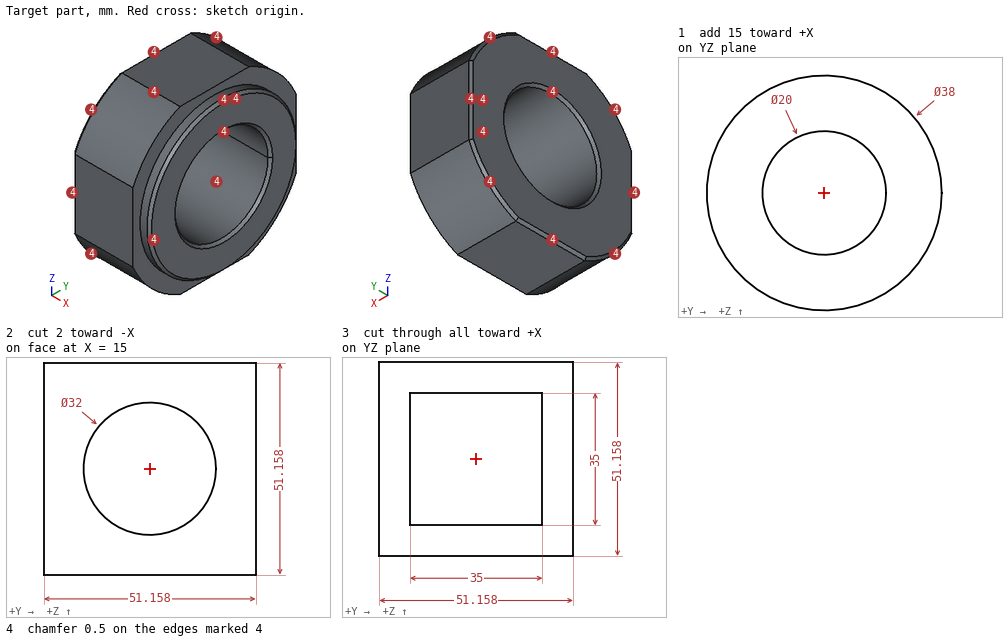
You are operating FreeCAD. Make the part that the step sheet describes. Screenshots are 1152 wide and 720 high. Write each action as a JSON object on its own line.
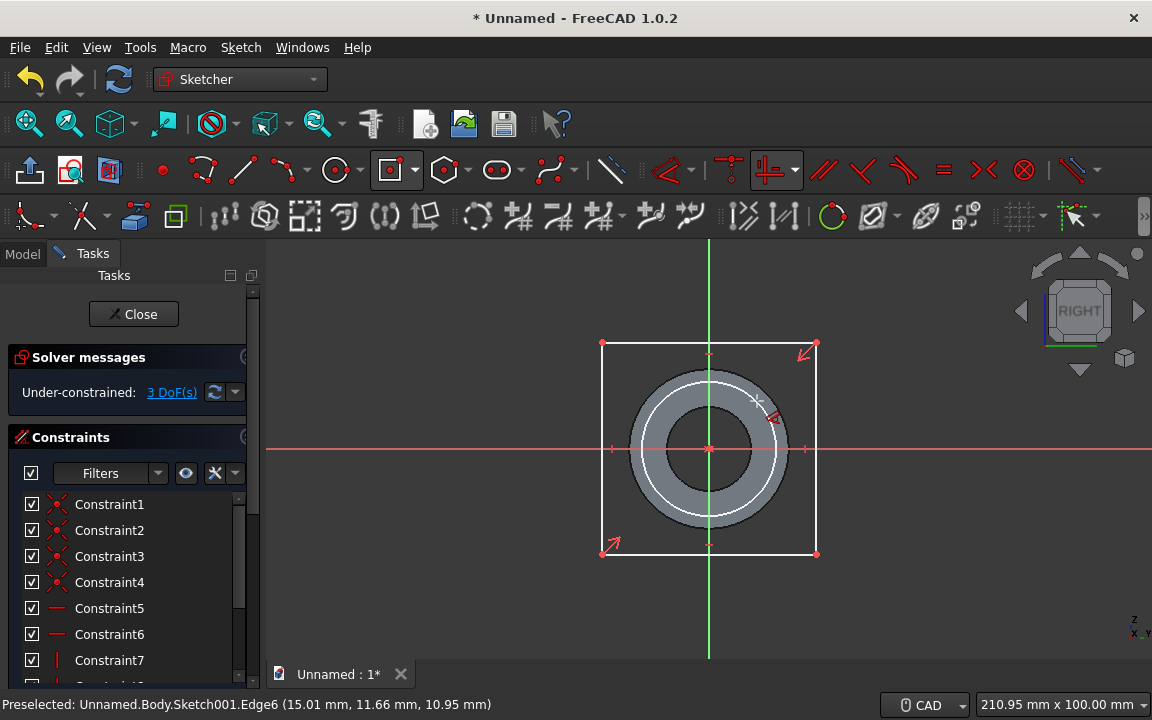
{"action": "left_click", "coordinate": [756, 401]}
{"action": "left_click", "coordinate": [778, 378]}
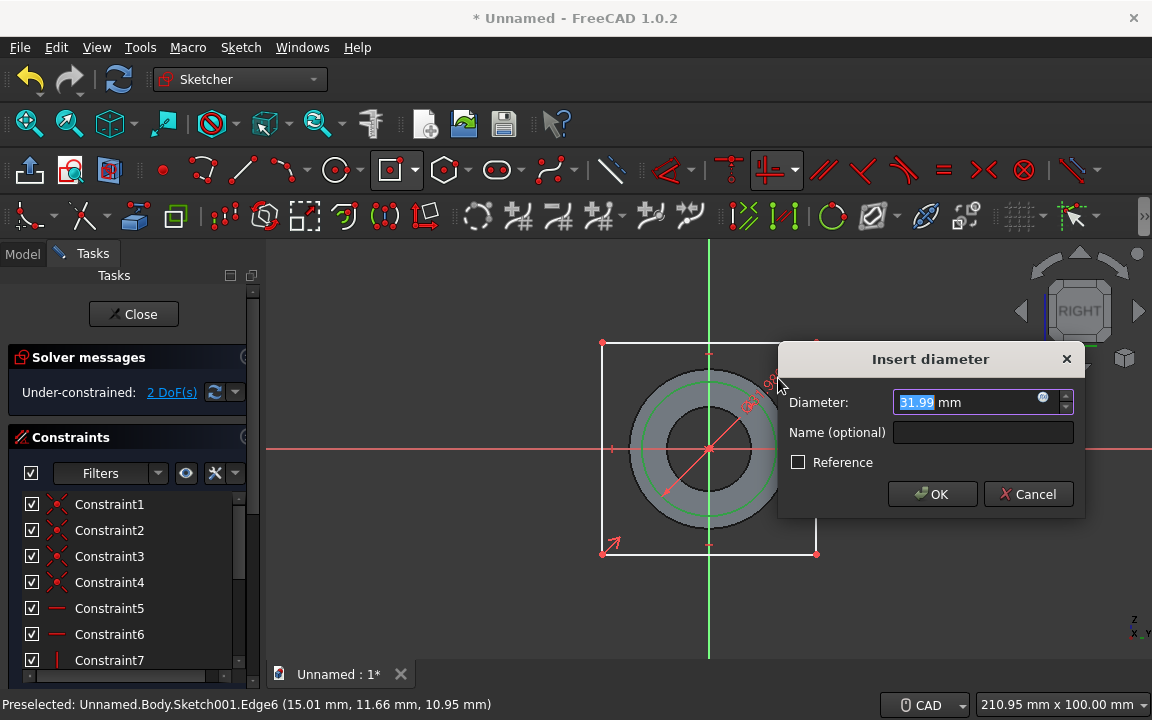
{"action": "type", "text": "32"}
{"action": "key", "text": "Return"}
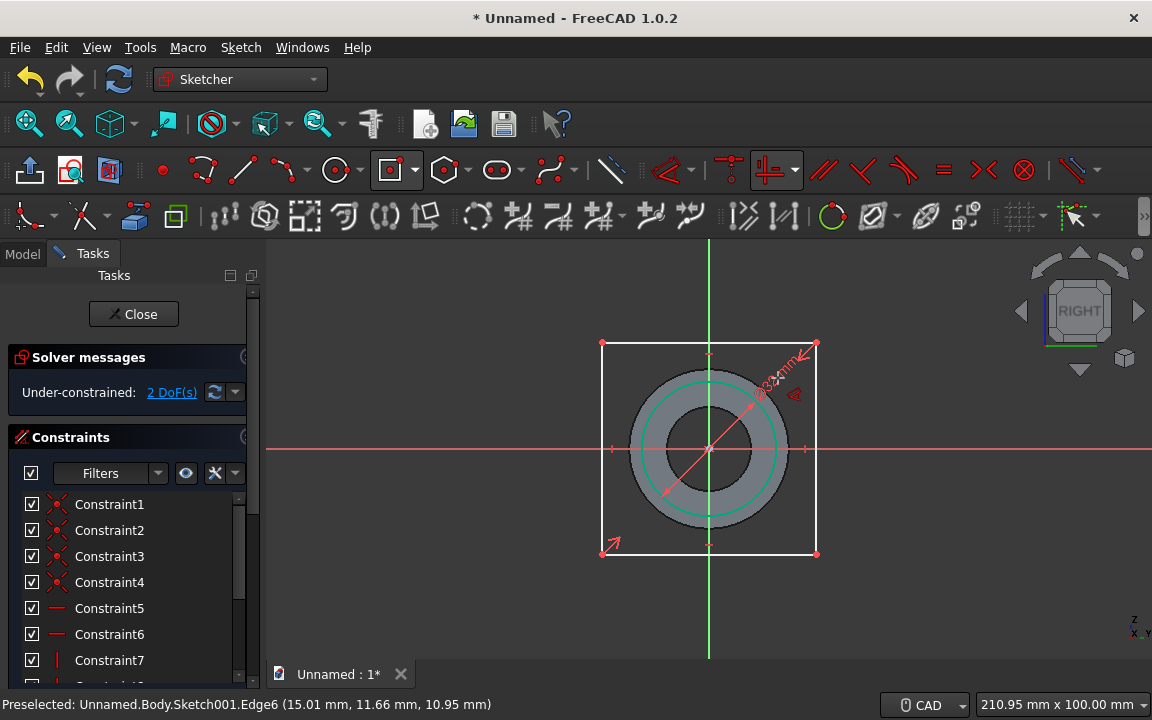
{"action": "left_click", "coordinate": [666, 555]}
{"action": "left_click", "coordinate": [660, 589]}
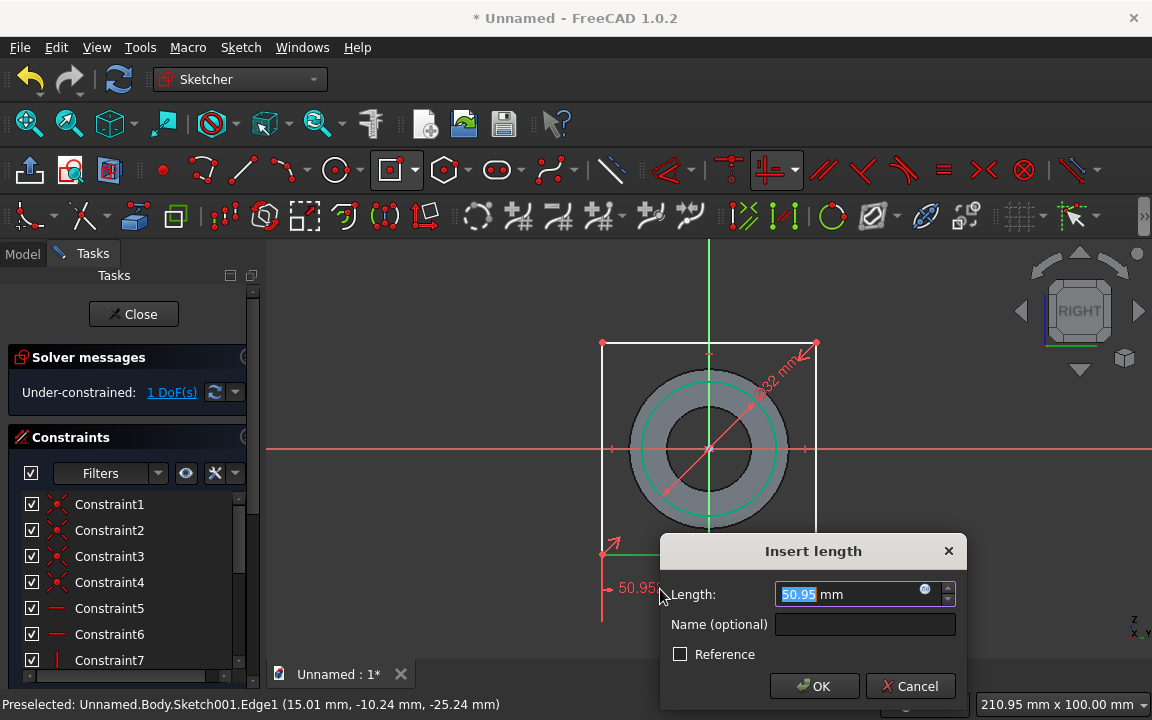
{"action": "type", "text": "51.158"}
{"action": "key", "text": "Return"}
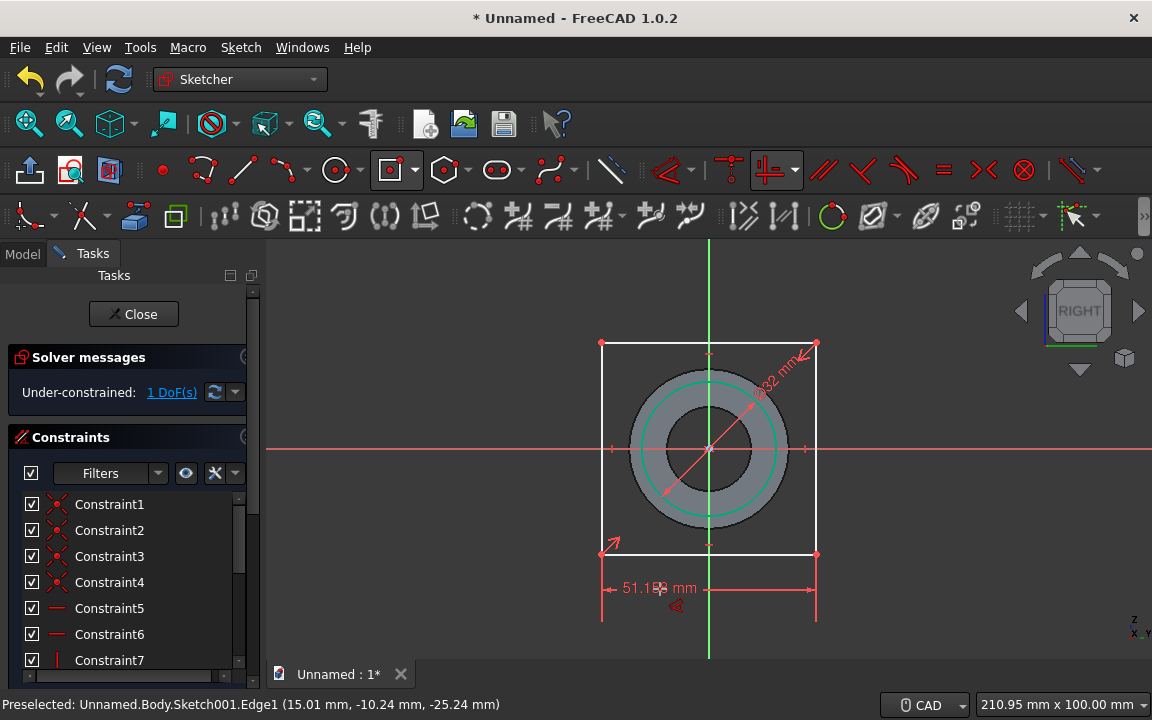
{"action": "left_click", "coordinate": [816, 491]}
{"action": "left_click", "coordinate": [850, 400]}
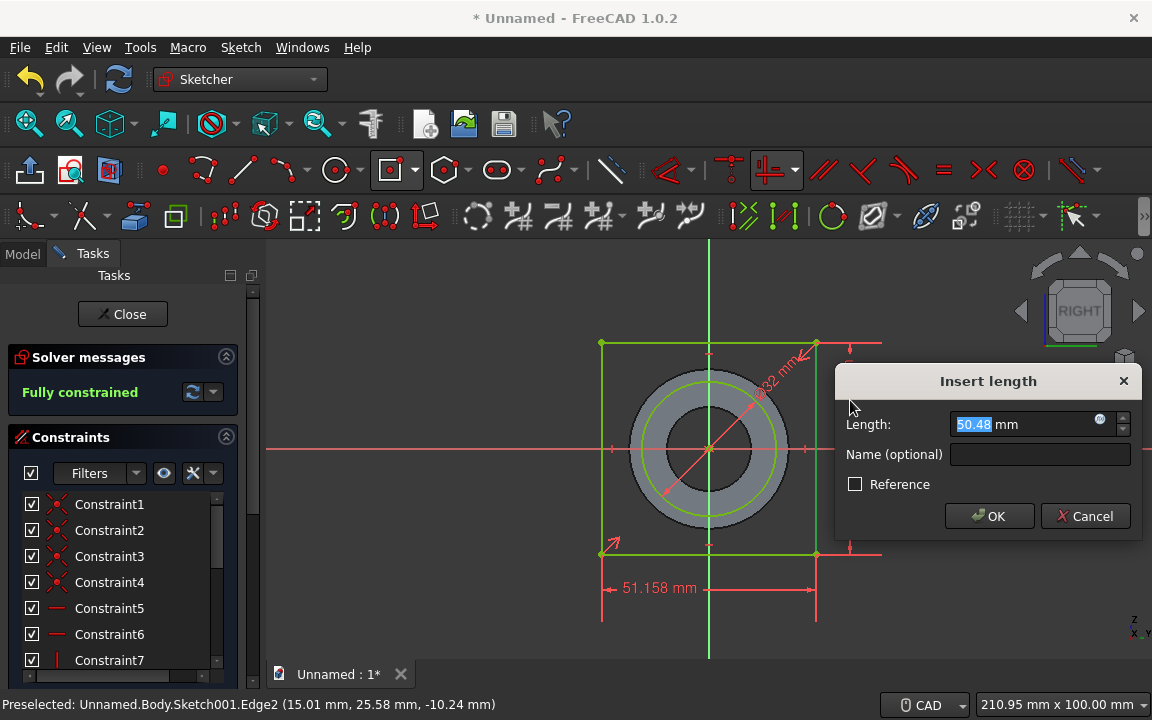
{"action": "type", "text": "51.158"}
{"action": "key", "text": "Return"}
{"action": "key", "text": "Escape"}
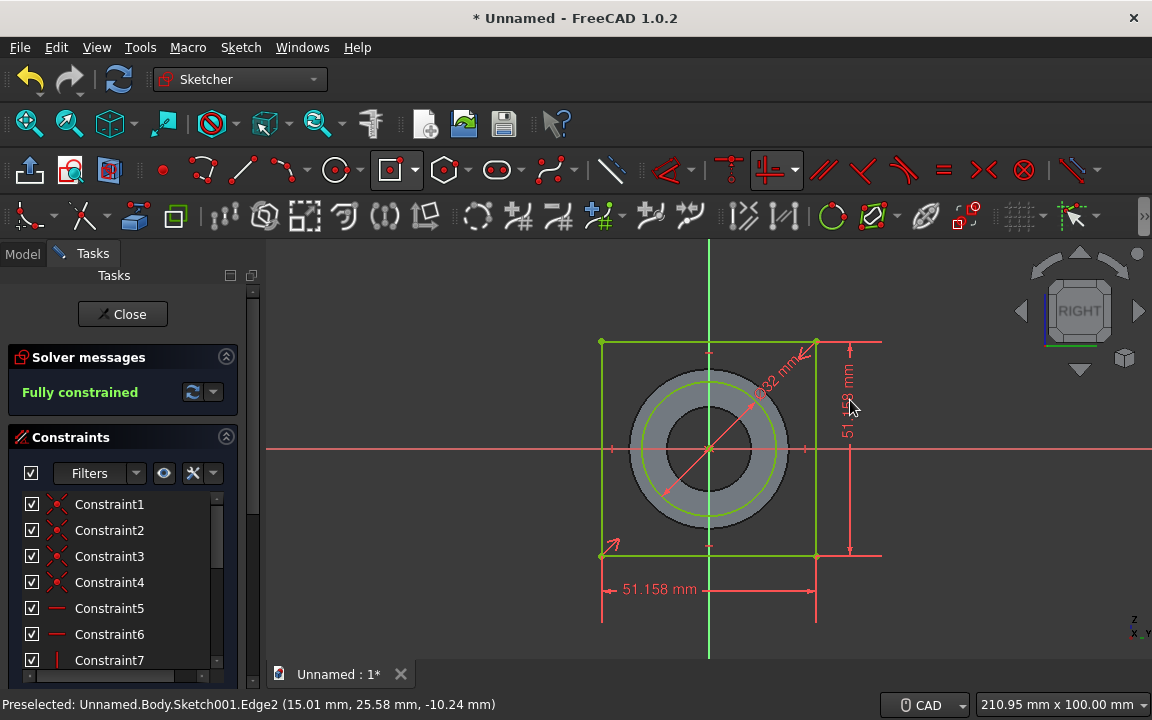
{"action": "left_click", "coordinate": [123, 314]}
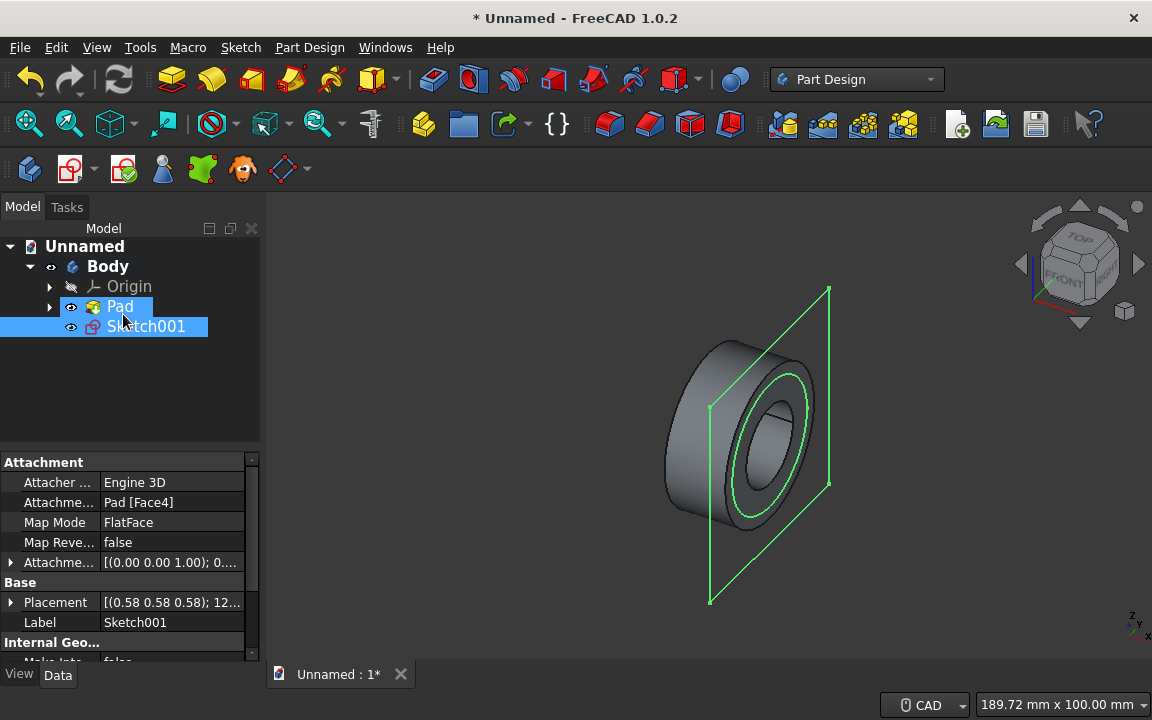
{"action": "left_click", "coordinate": [434, 80]}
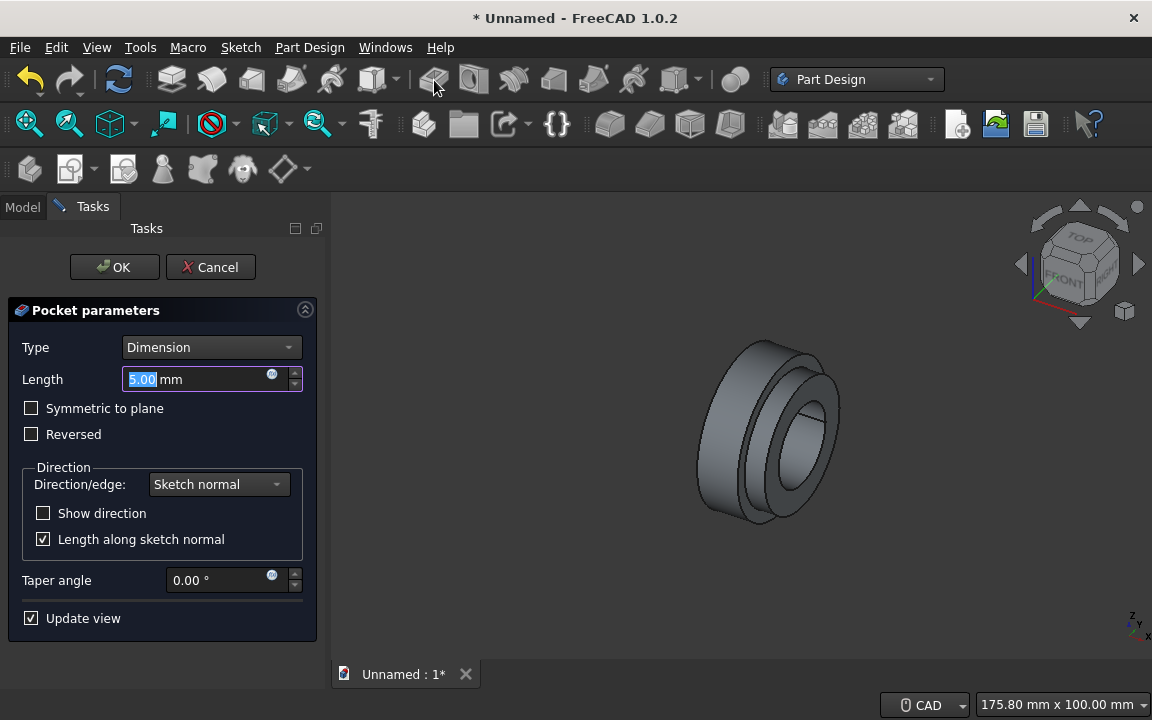
{"action": "type", "text": "2"}
{"action": "key", "text": "Tab"}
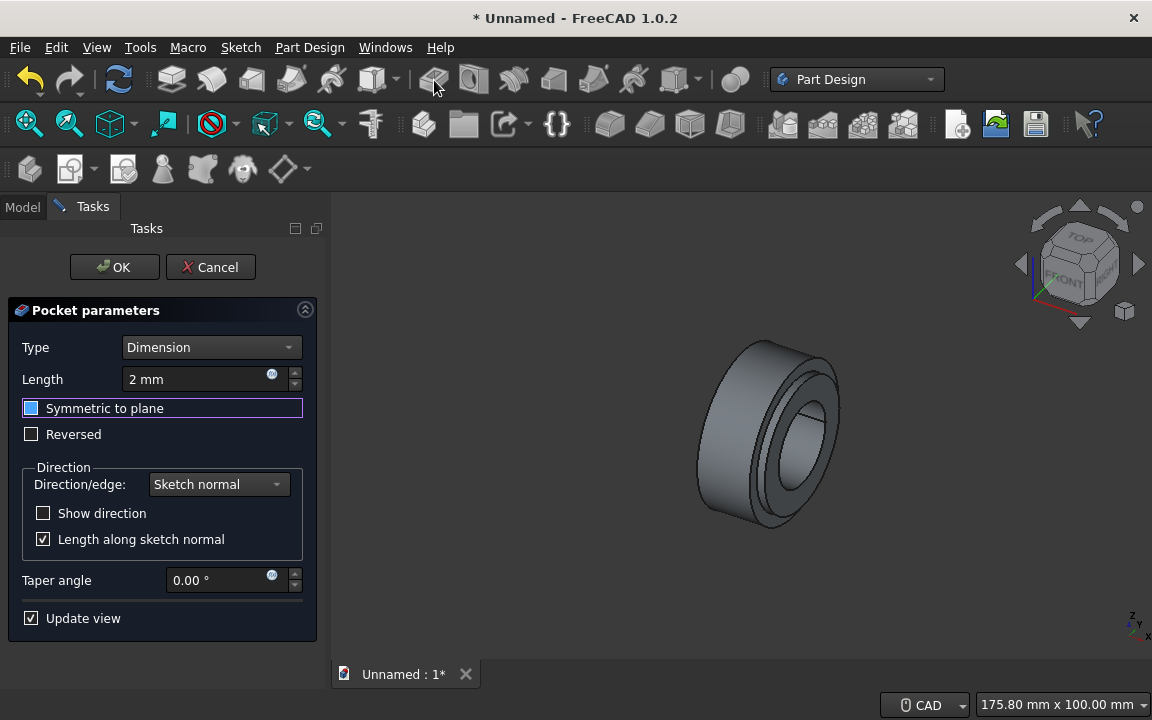
{"action": "left_click", "coordinate": [115, 267]}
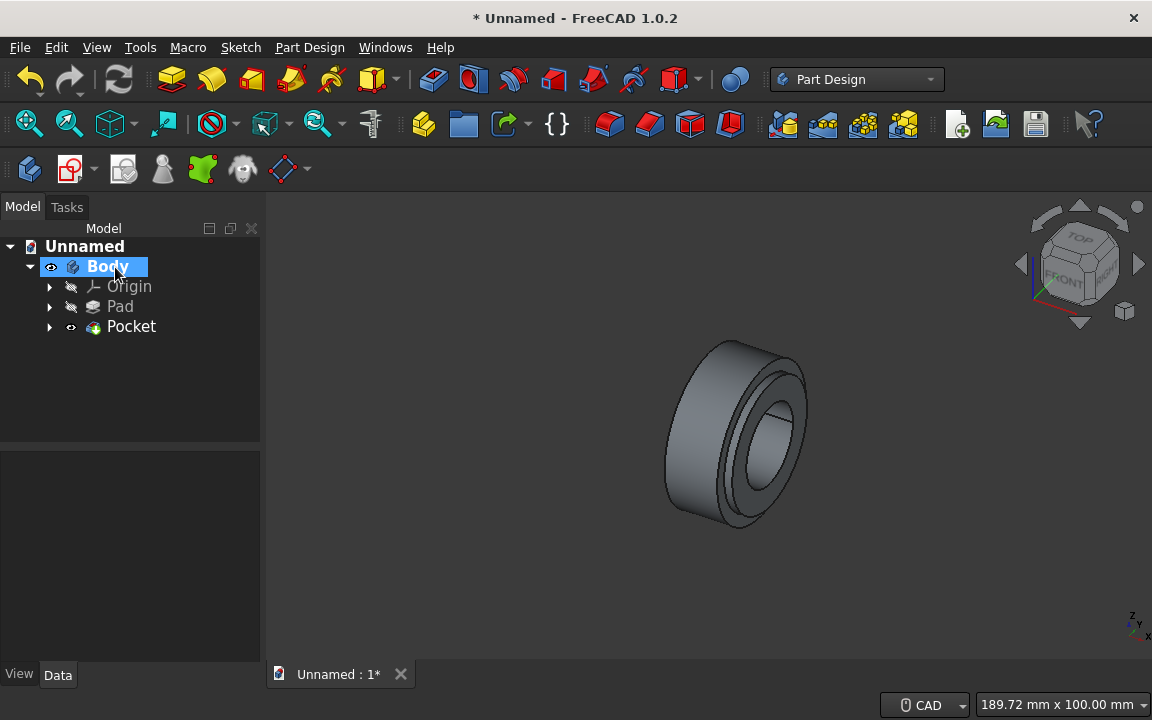
{"action": "left_click", "coordinate": [70, 170]}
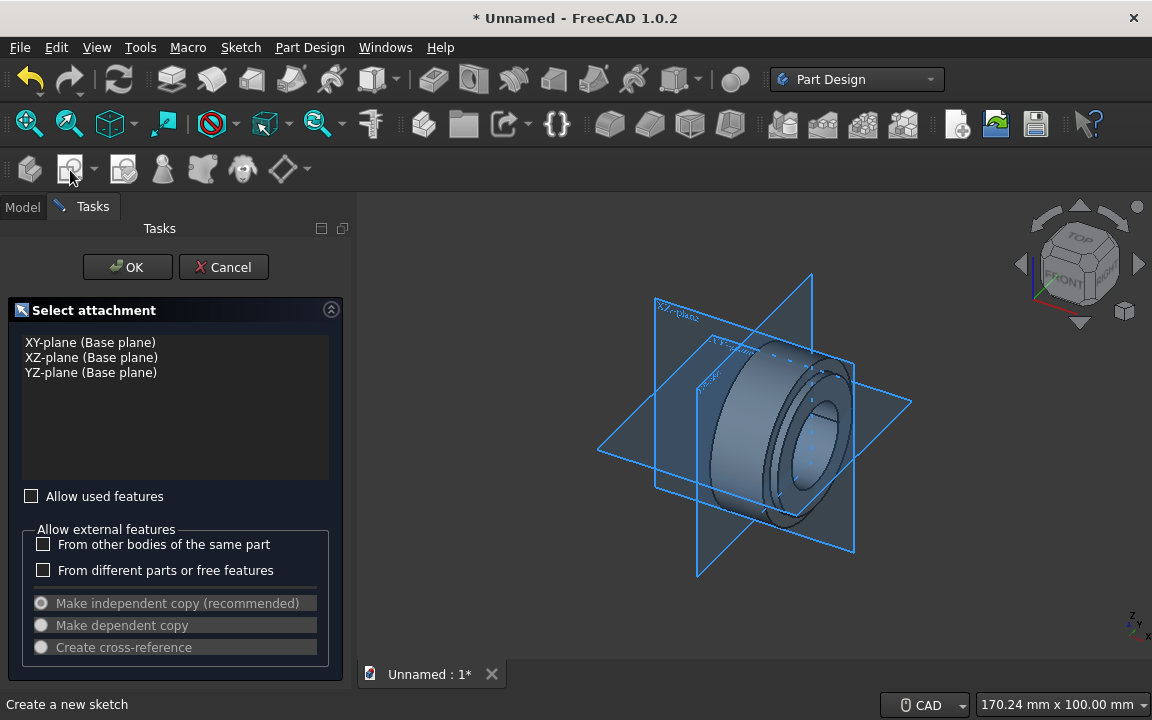
{"action": "left_click", "coordinate": [82, 372]}